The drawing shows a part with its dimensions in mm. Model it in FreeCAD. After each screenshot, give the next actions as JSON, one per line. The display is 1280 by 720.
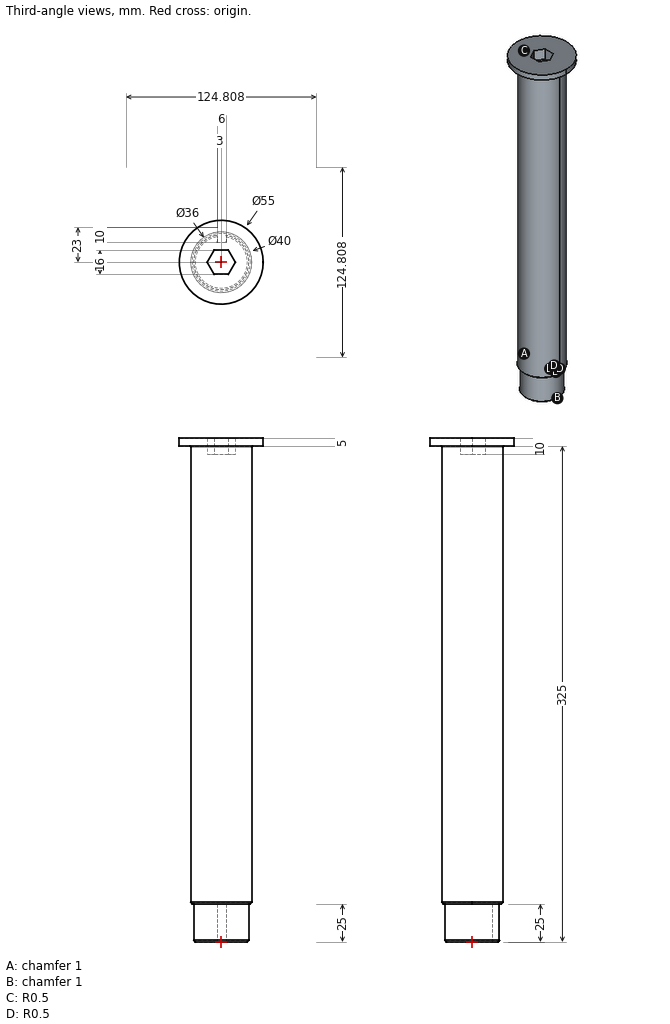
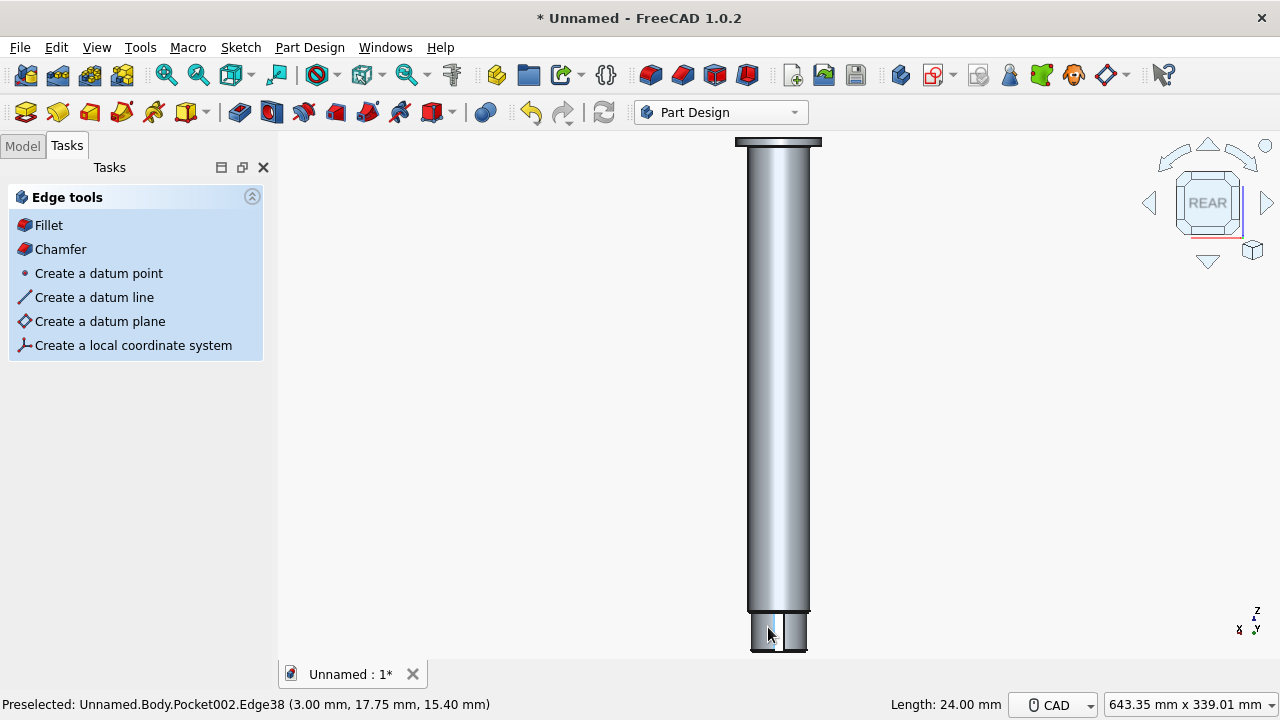
{"action": "left_click", "coordinate": [784, 627], "text": "ctrl"}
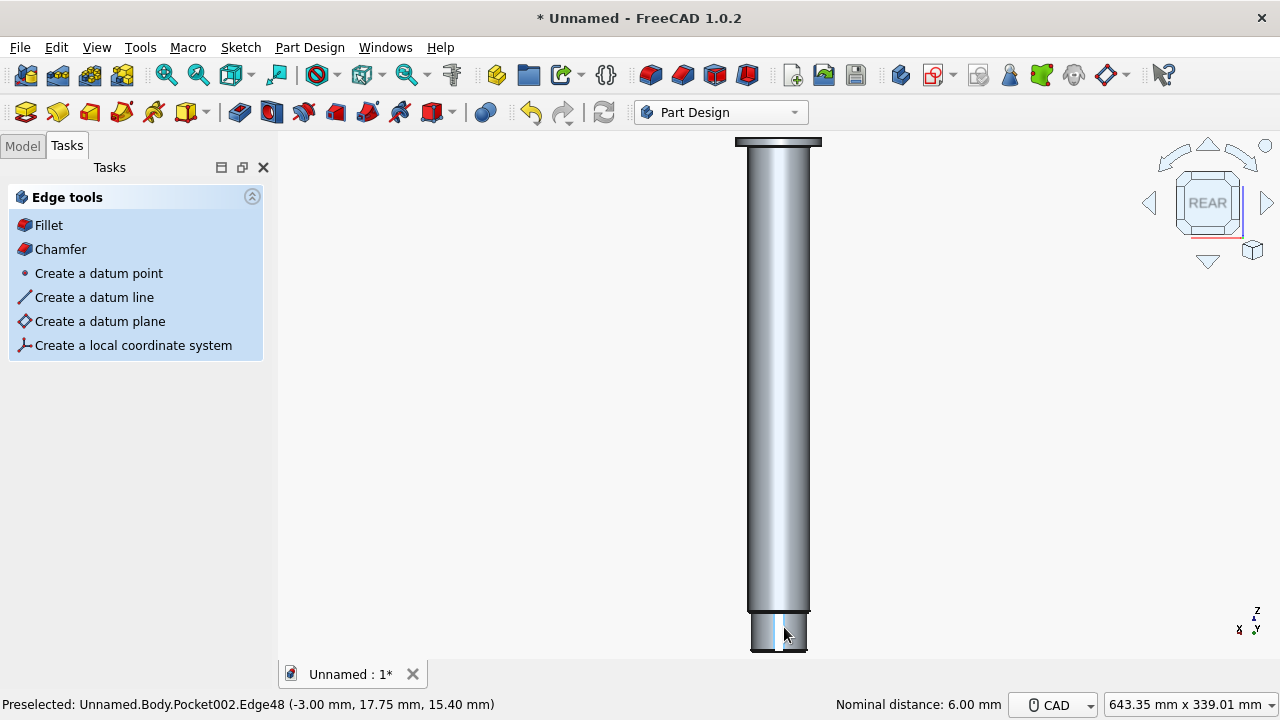
{"action": "key", "text": "6"}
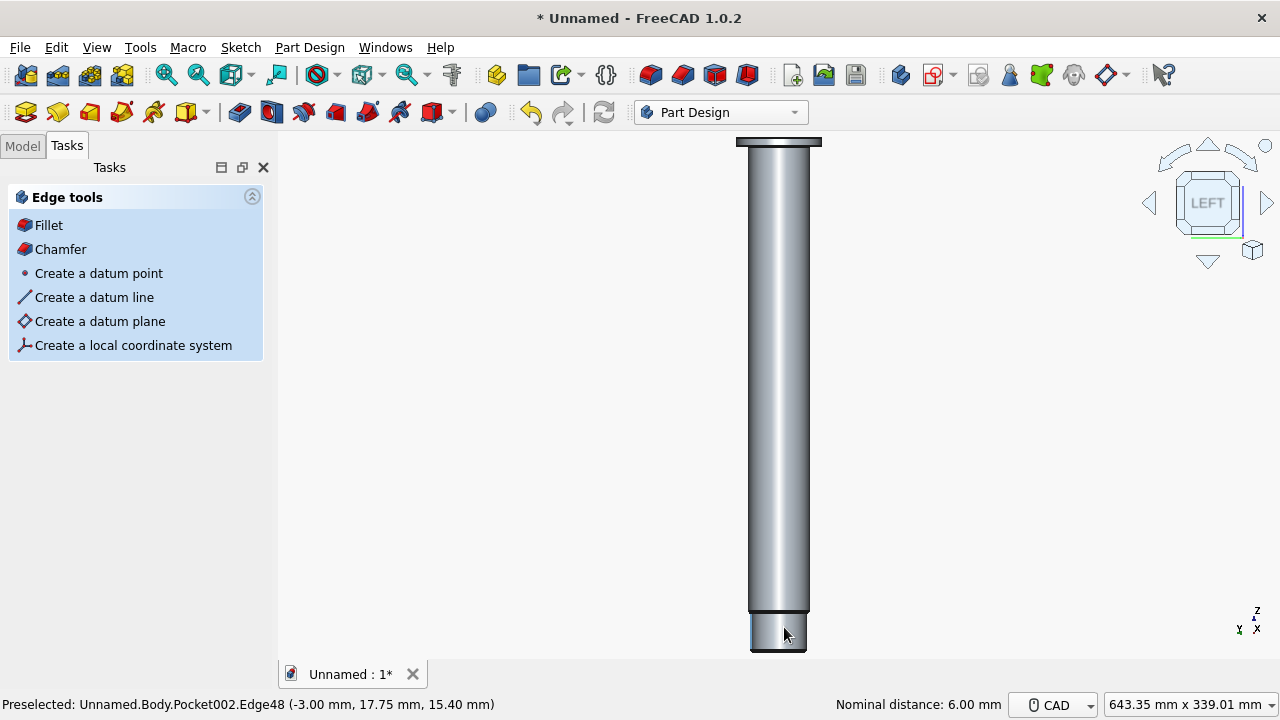
{"action": "key", "text": "v 3"}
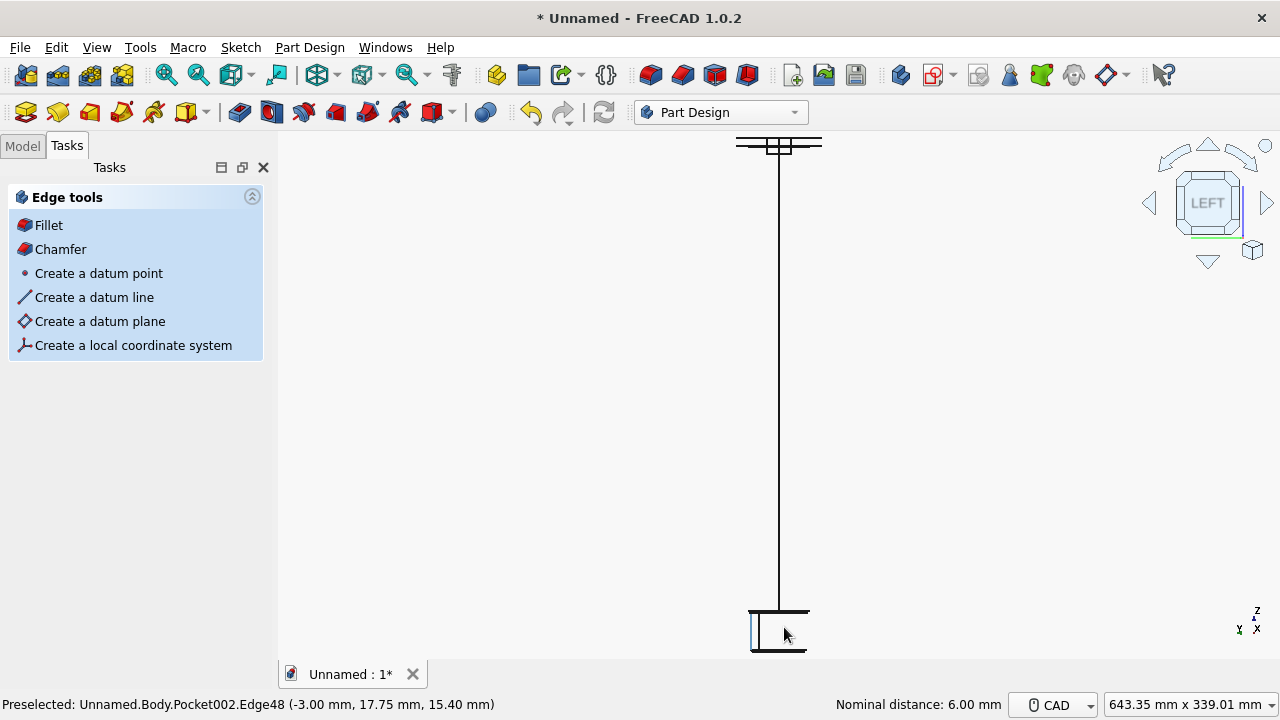
{"action": "key", "text": "0"}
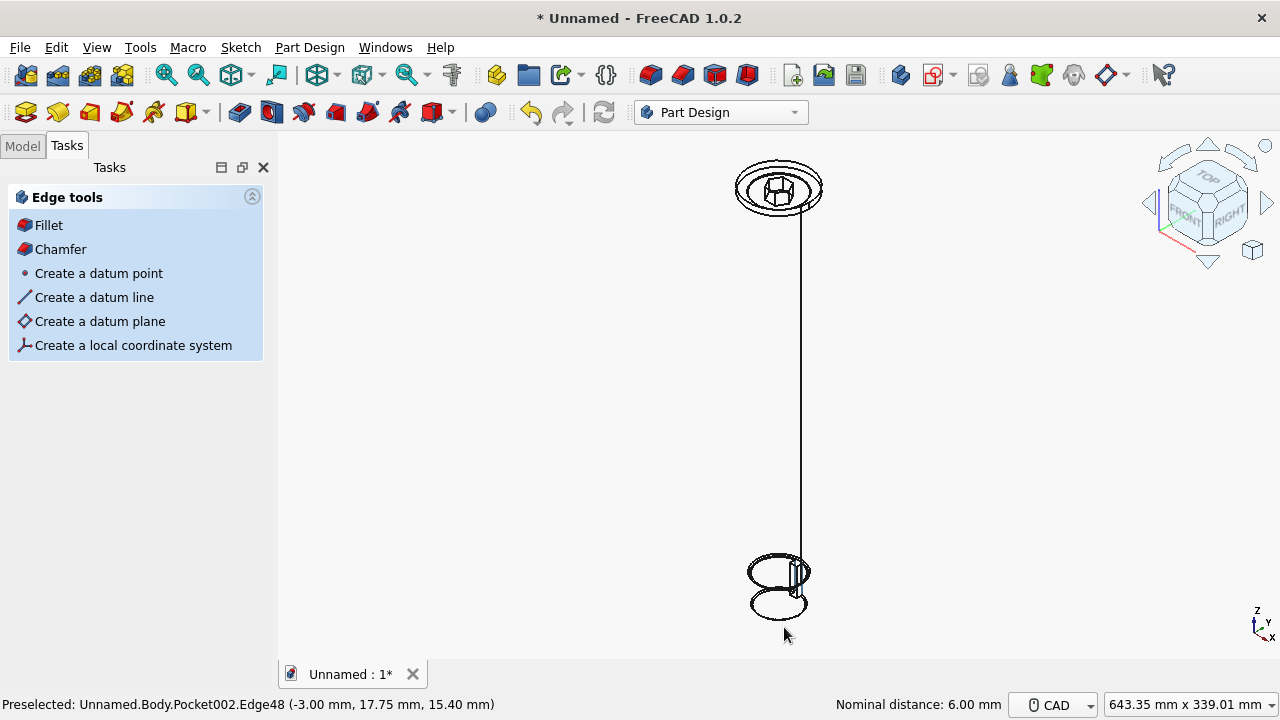
{"action": "left_click", "coordinate": [790, 578], "text": "ctrl"}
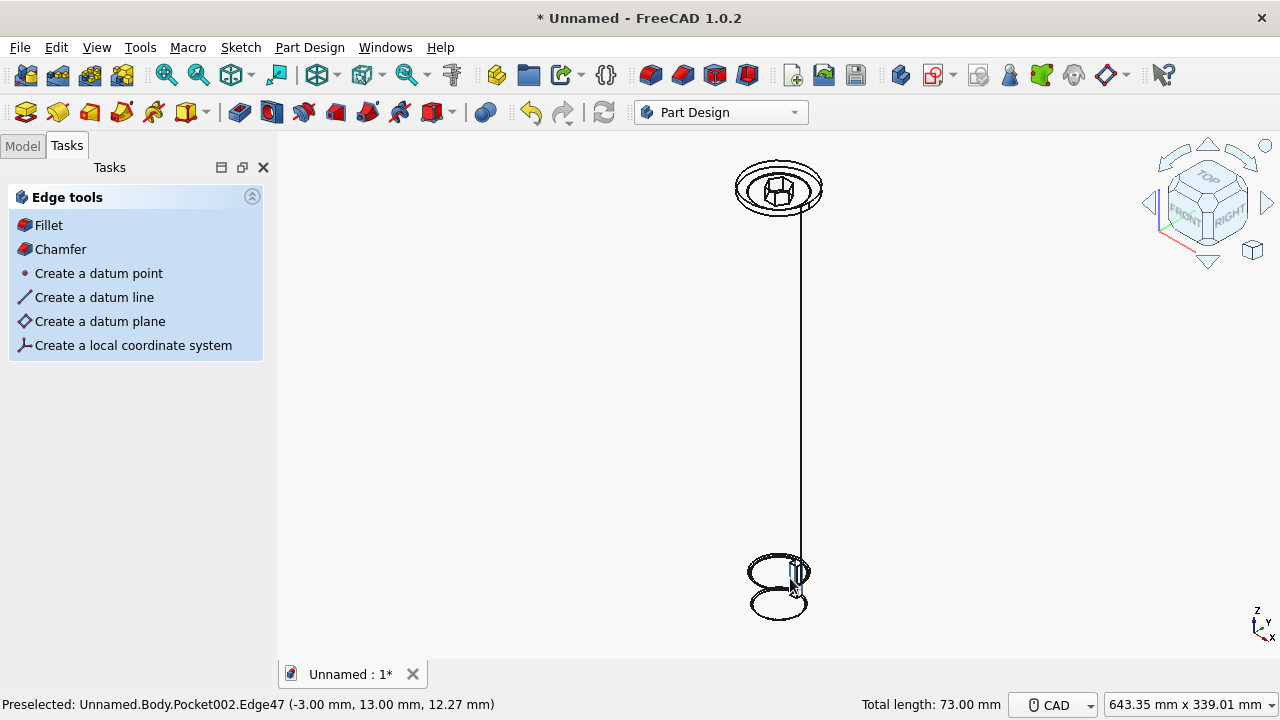
{"action": "left_click", "coordinate": [797, 594], "text": "ctrl"}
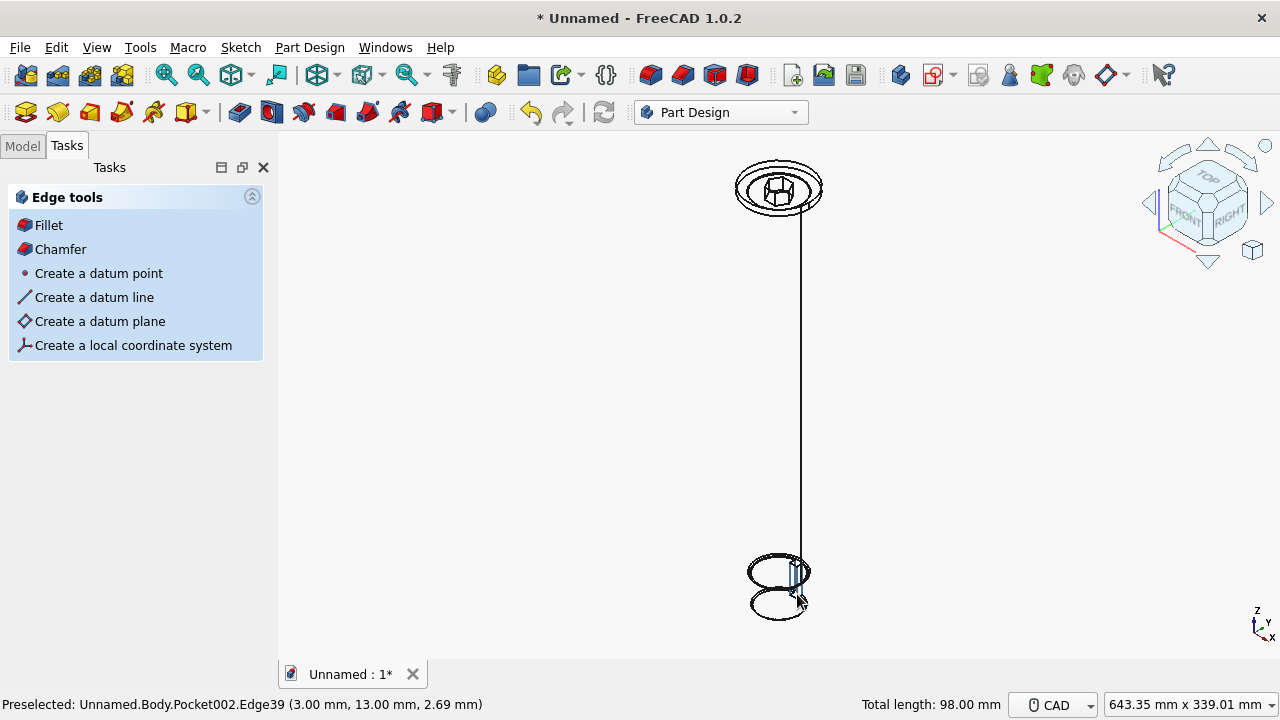
{"action": "key", "text": "v 1"}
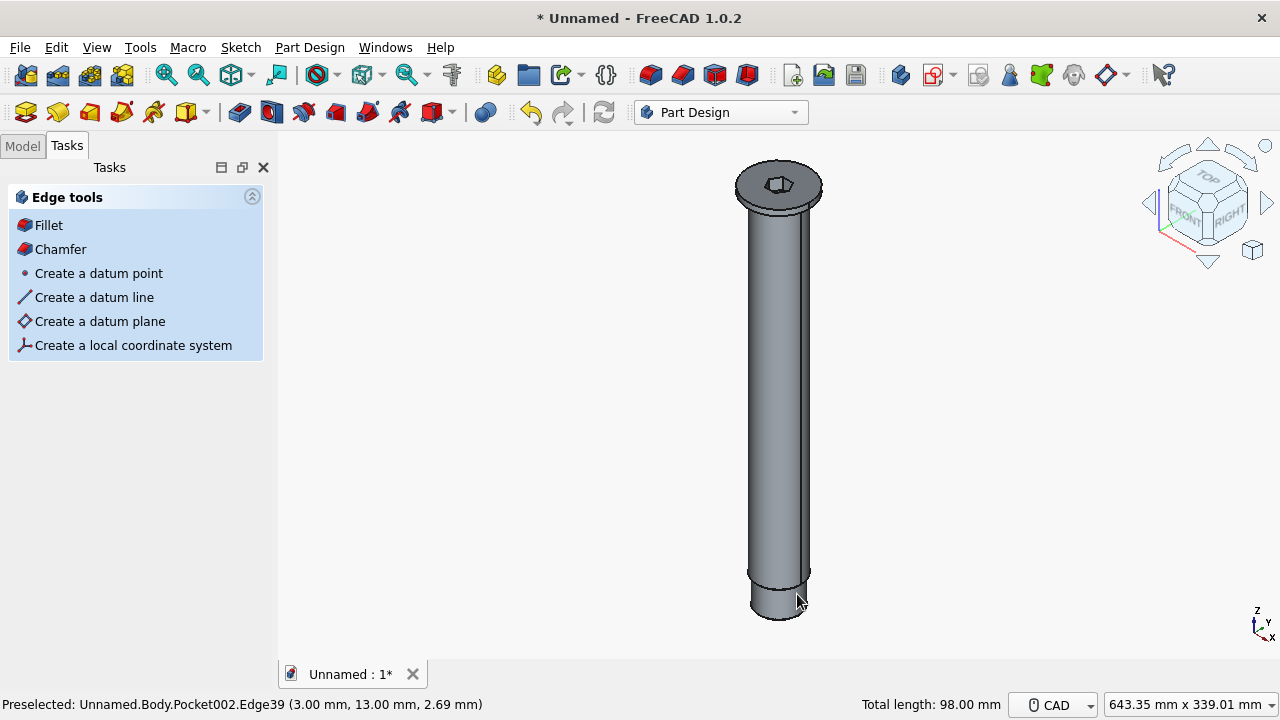
{"action": "left_click", "coordinate": [652, 76]}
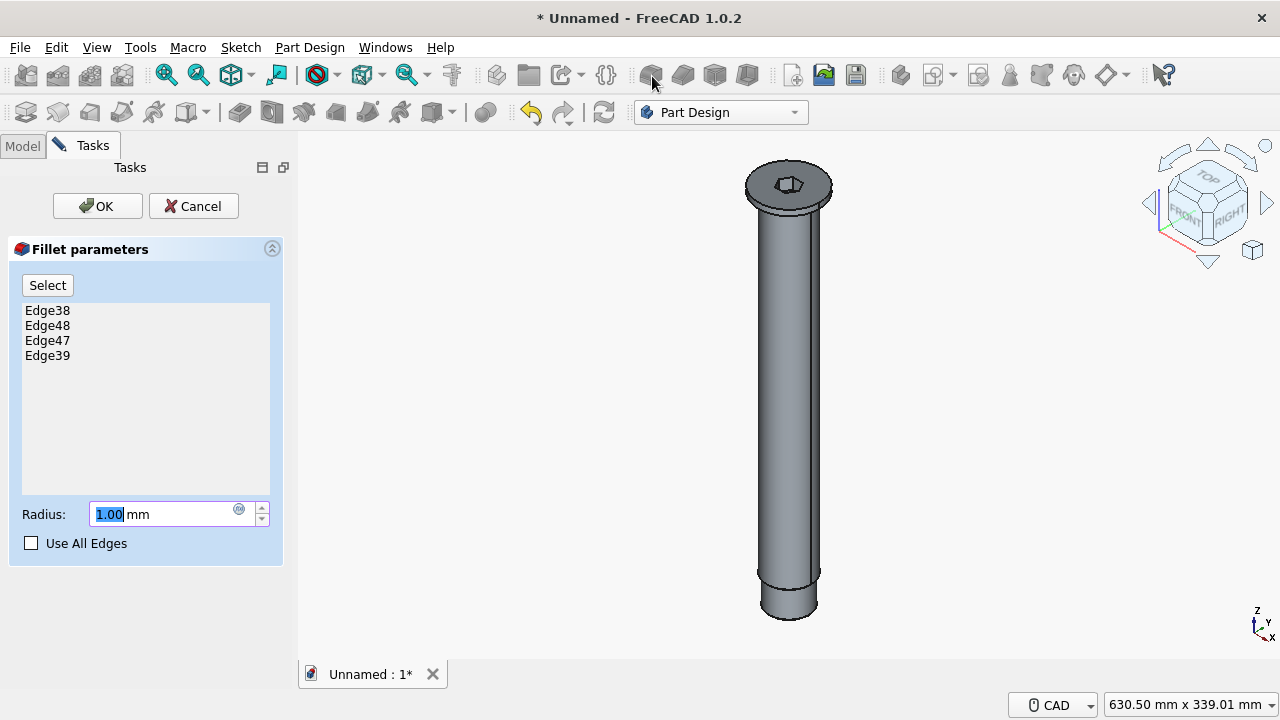
{"action": "type", "text": "0.5"}
{"action": "key", "text": "Tab"}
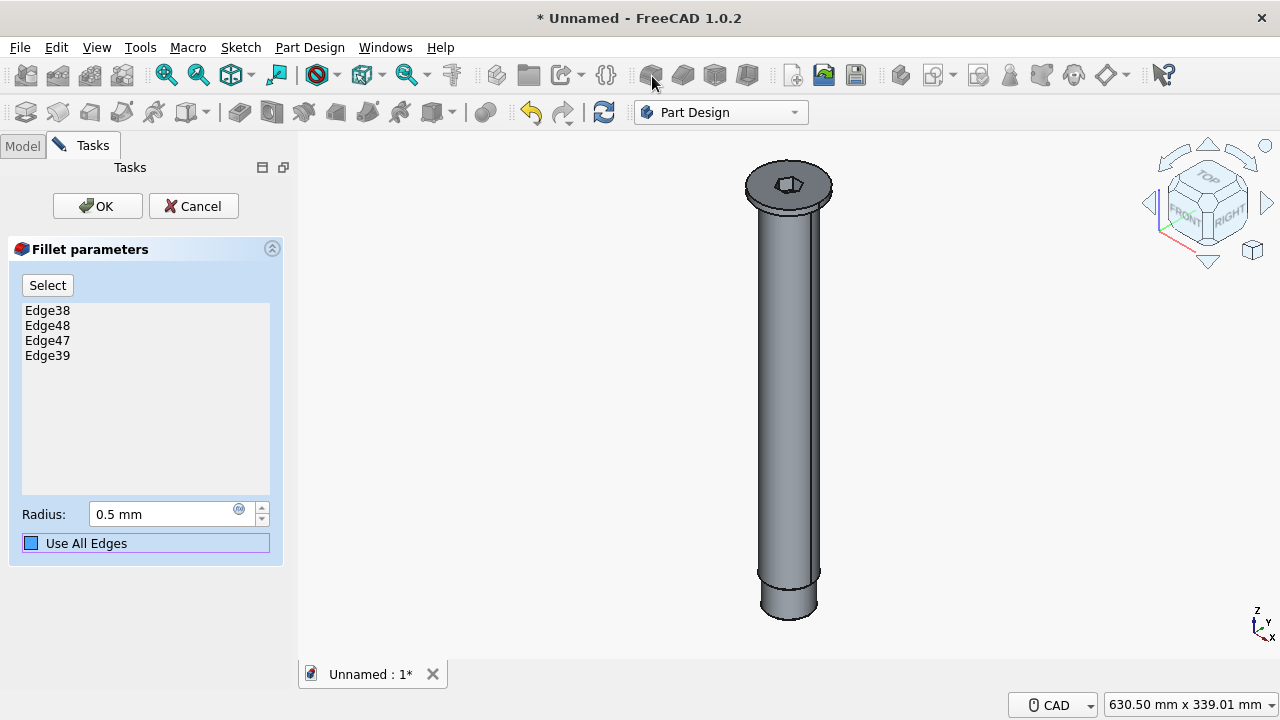
{"action": "left_click", "coordinate": [98, 206]}